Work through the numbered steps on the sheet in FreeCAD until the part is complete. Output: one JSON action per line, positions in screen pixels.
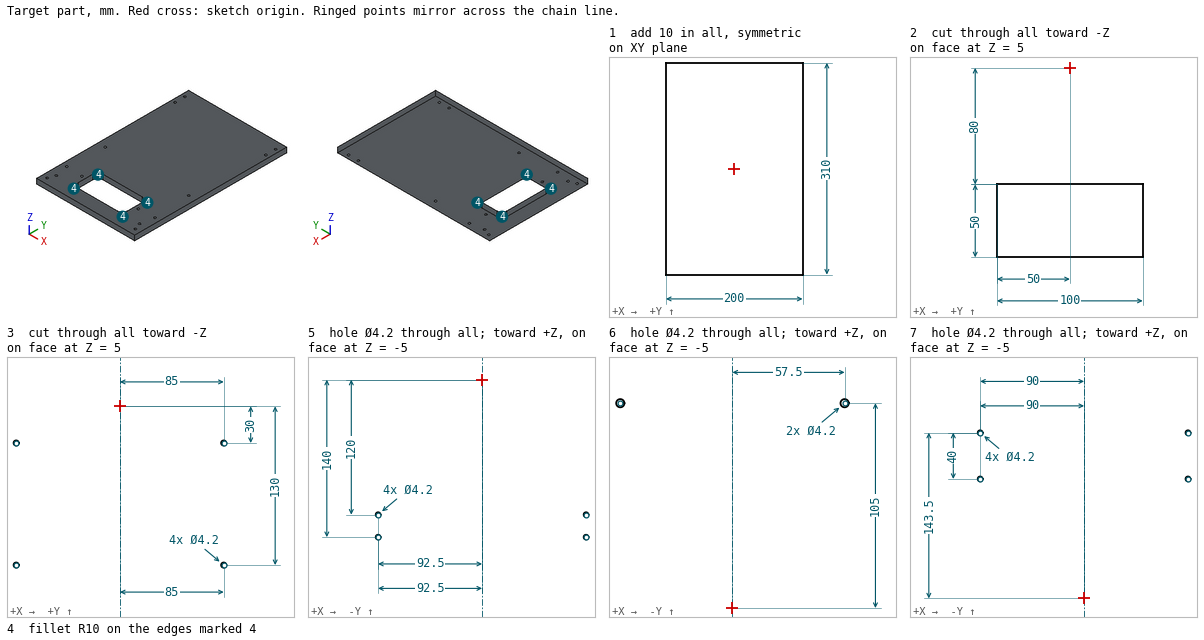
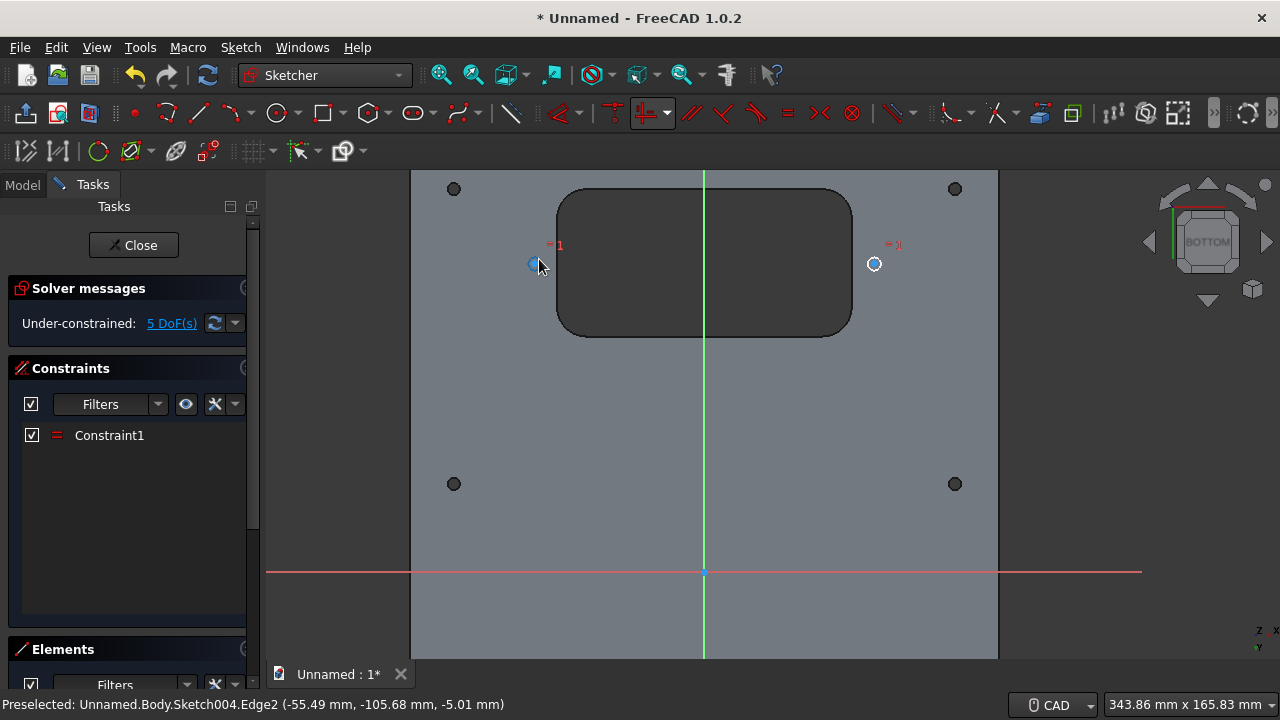
{"action": "left_click", "coordinate": [874, 264]}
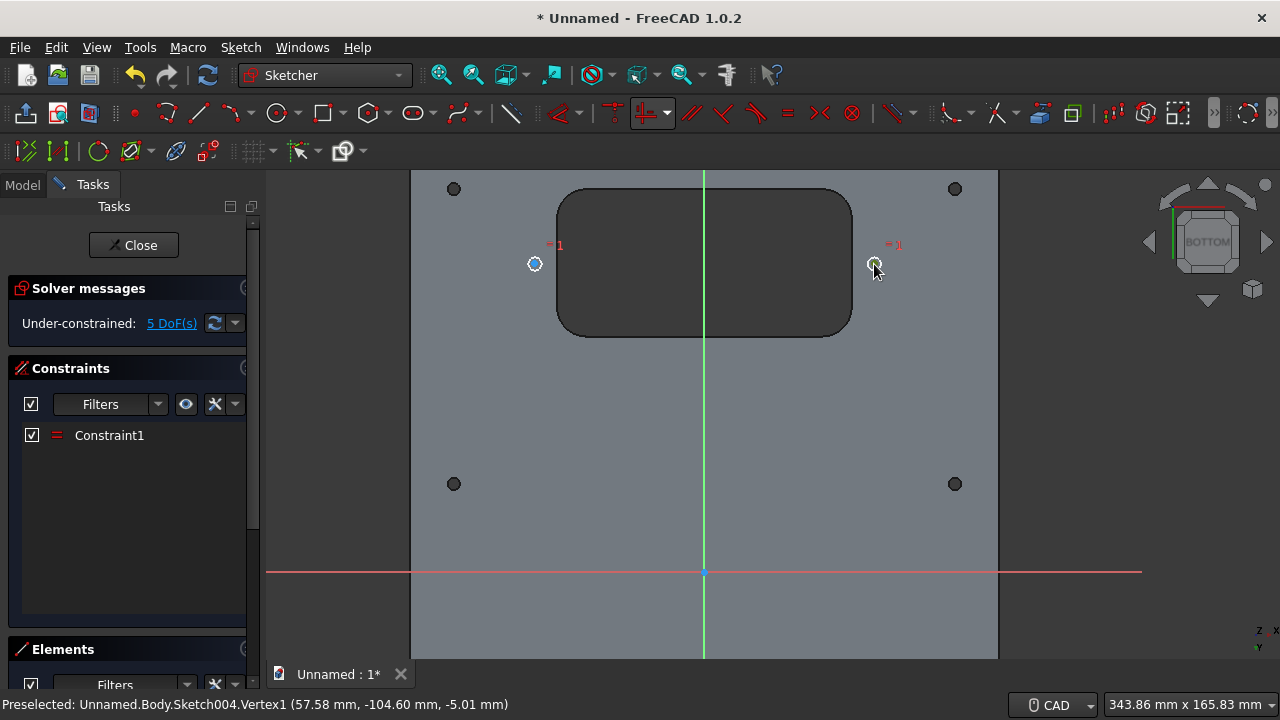
{"action": "left_click", "coordinate": [535, 264]}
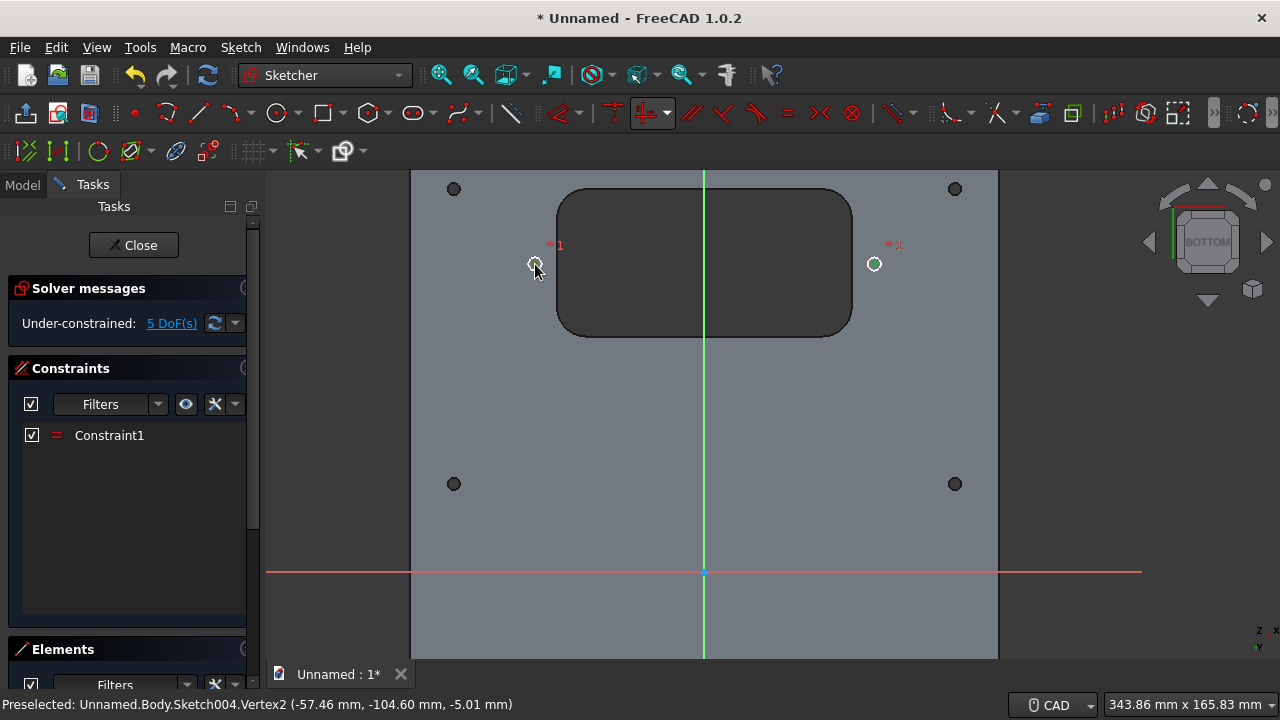
{"action": "left_click", "coordinate": [704, 538]}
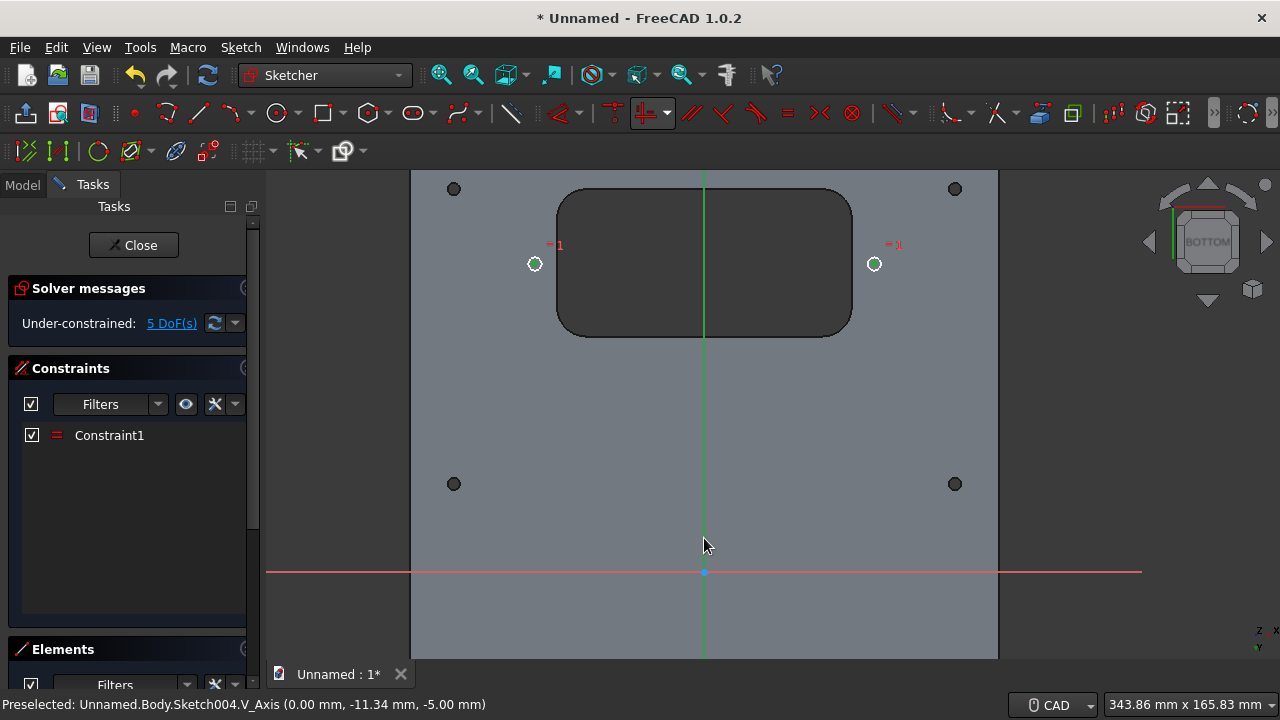
{"action": "left_click", "coordinate": [820, 114]}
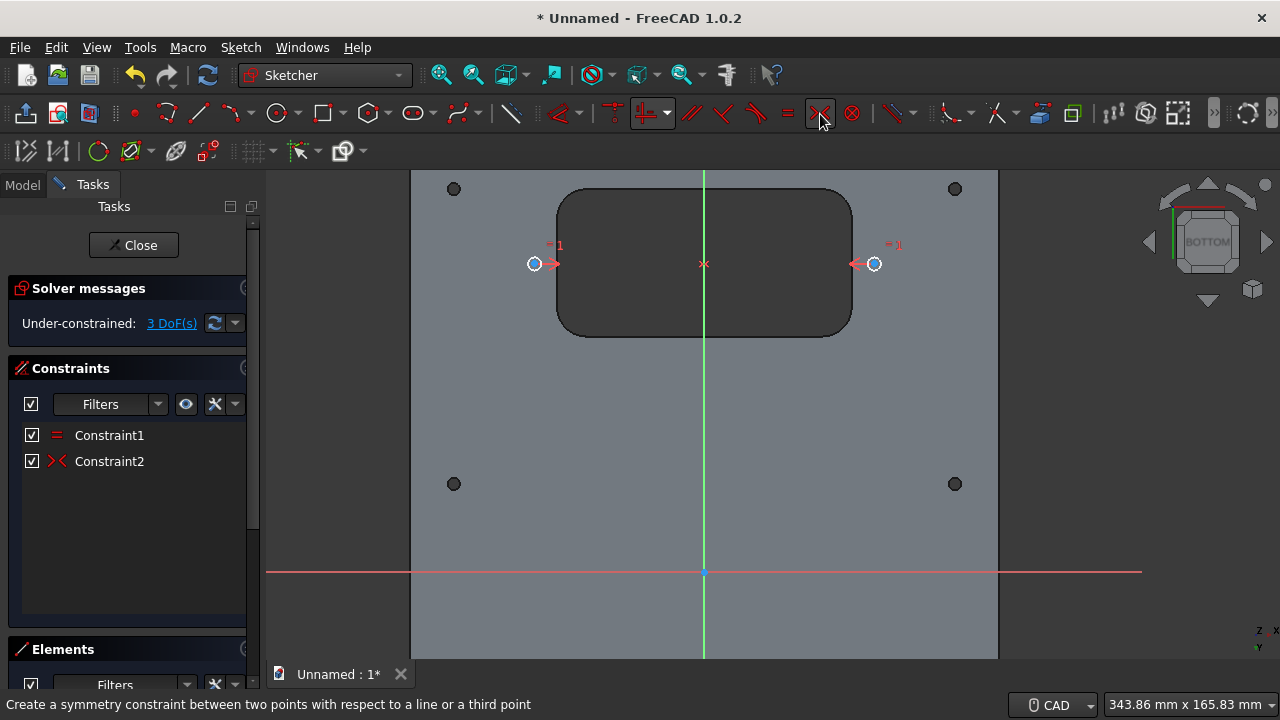
{"action": "left_click", "coordinate": [558, 114]}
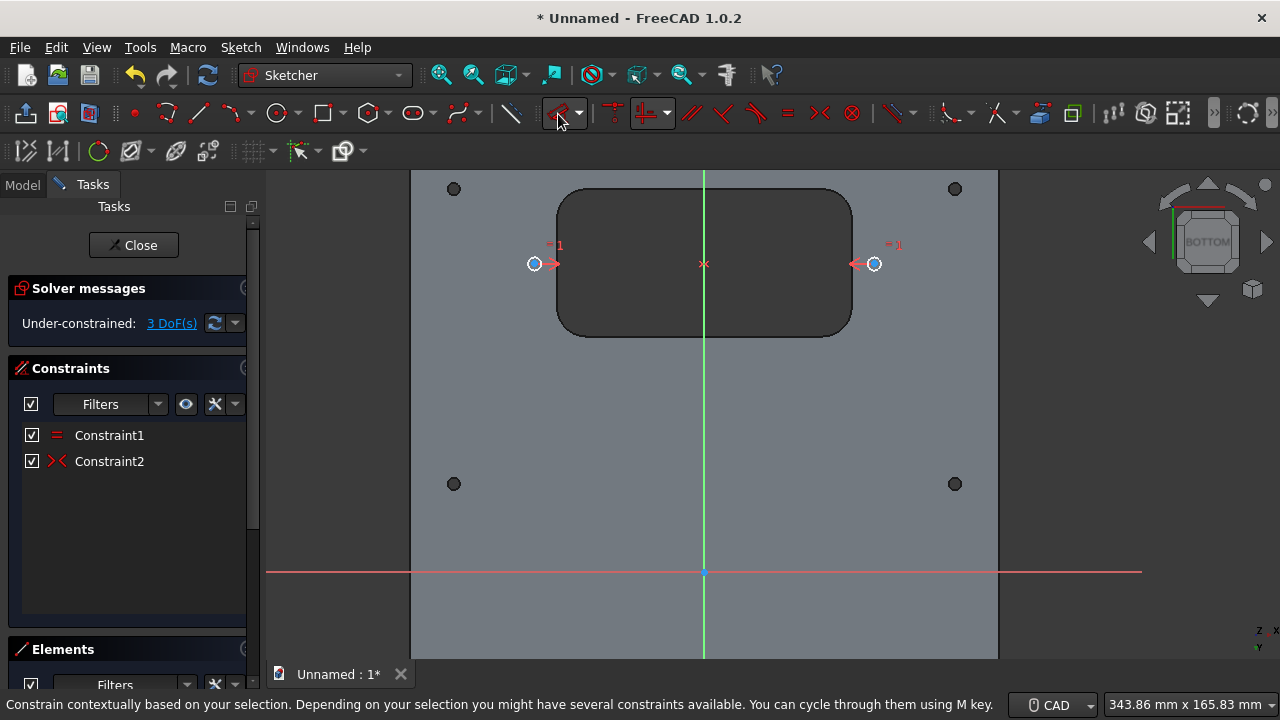
{"action": "scroll", "coordinate": [879, 259], "scroll_direction": "up", "scroll_amount": 6}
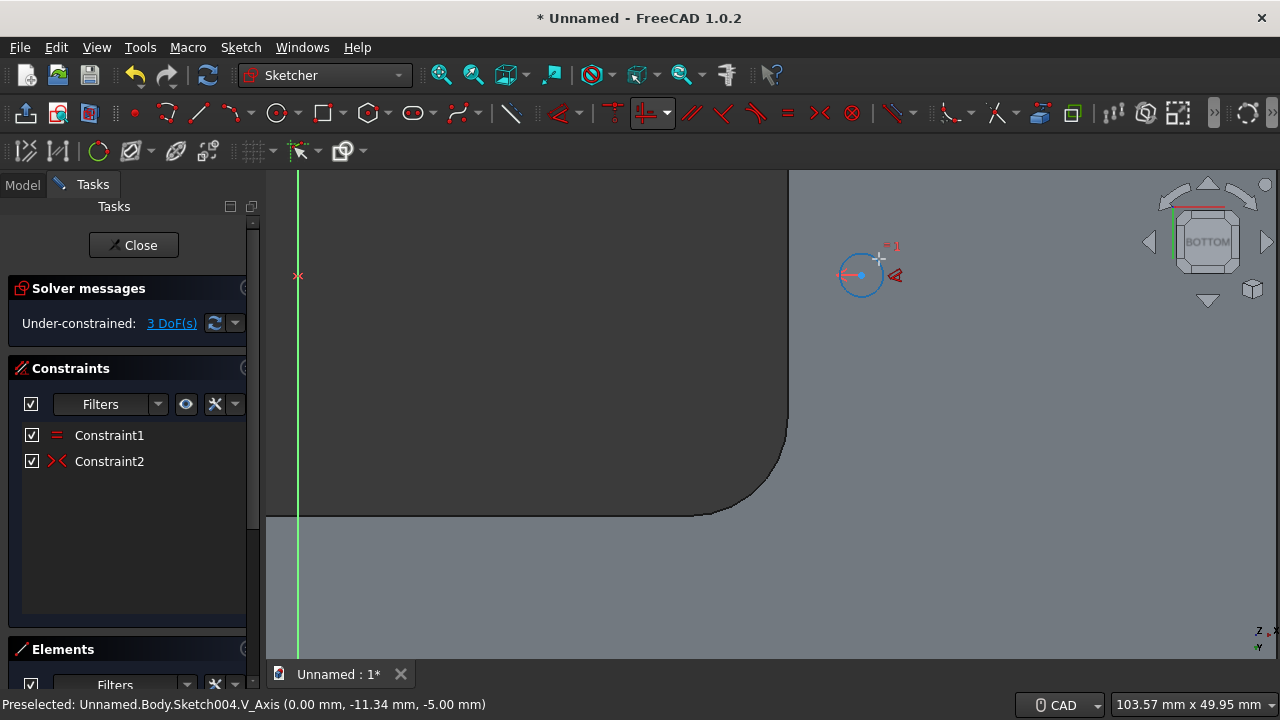
{"action": "left_click", "coordinate": [877, 260]}
{"action": "left_click", "coordinate": [900, 238]}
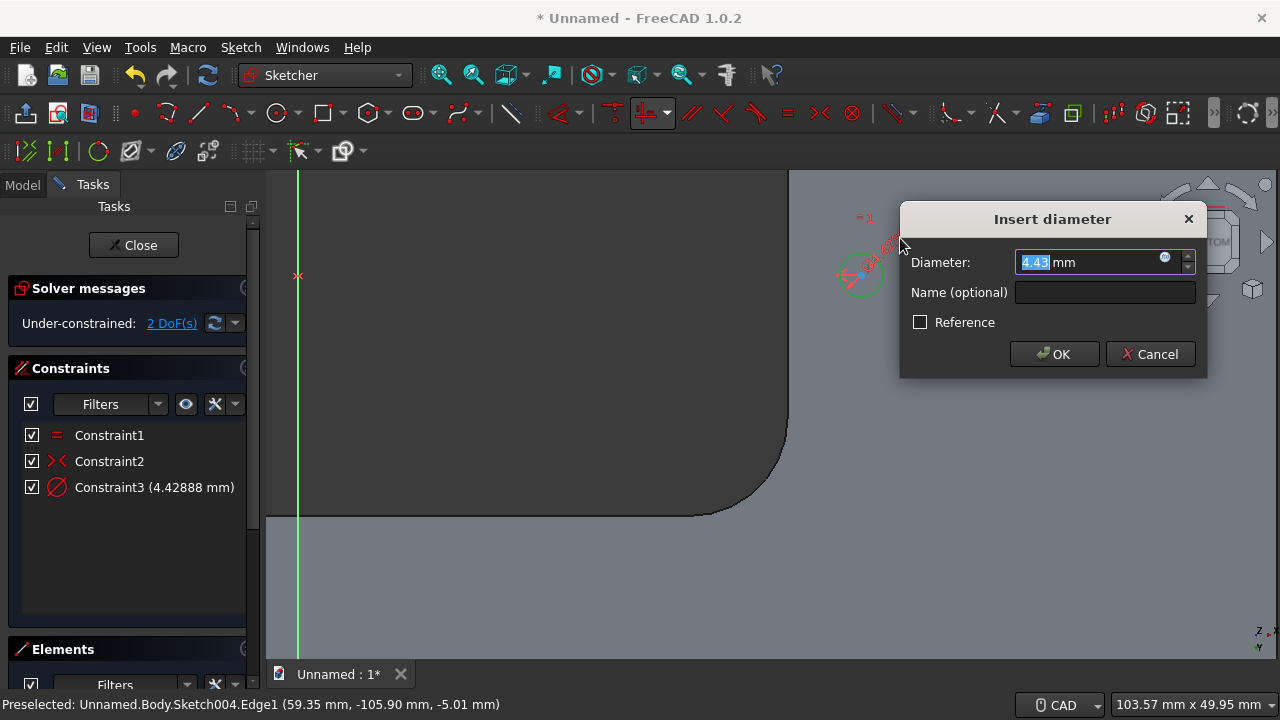
{"action": "type", "text": "4.2"}
{"action": "key", "text": "Return"}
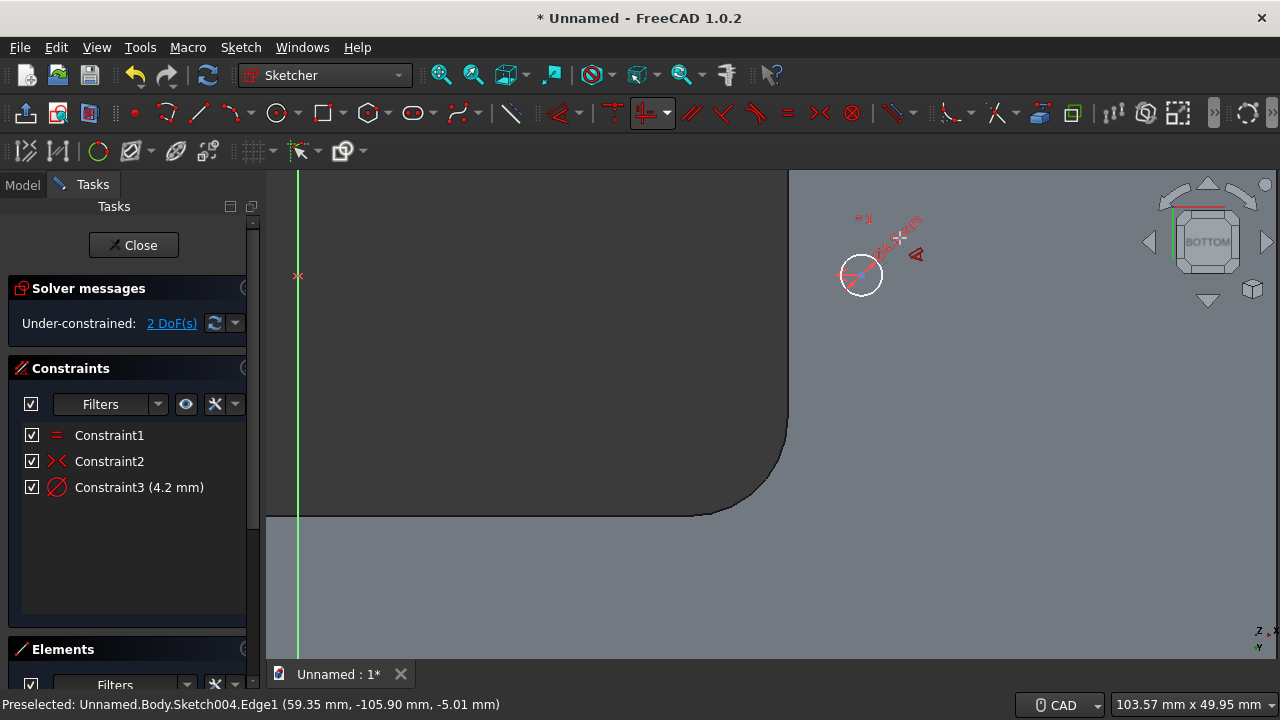
{"action": "left_click", "coordinate": [862, 275]}
{"action": "left_click", "coordinate": [896, 453]}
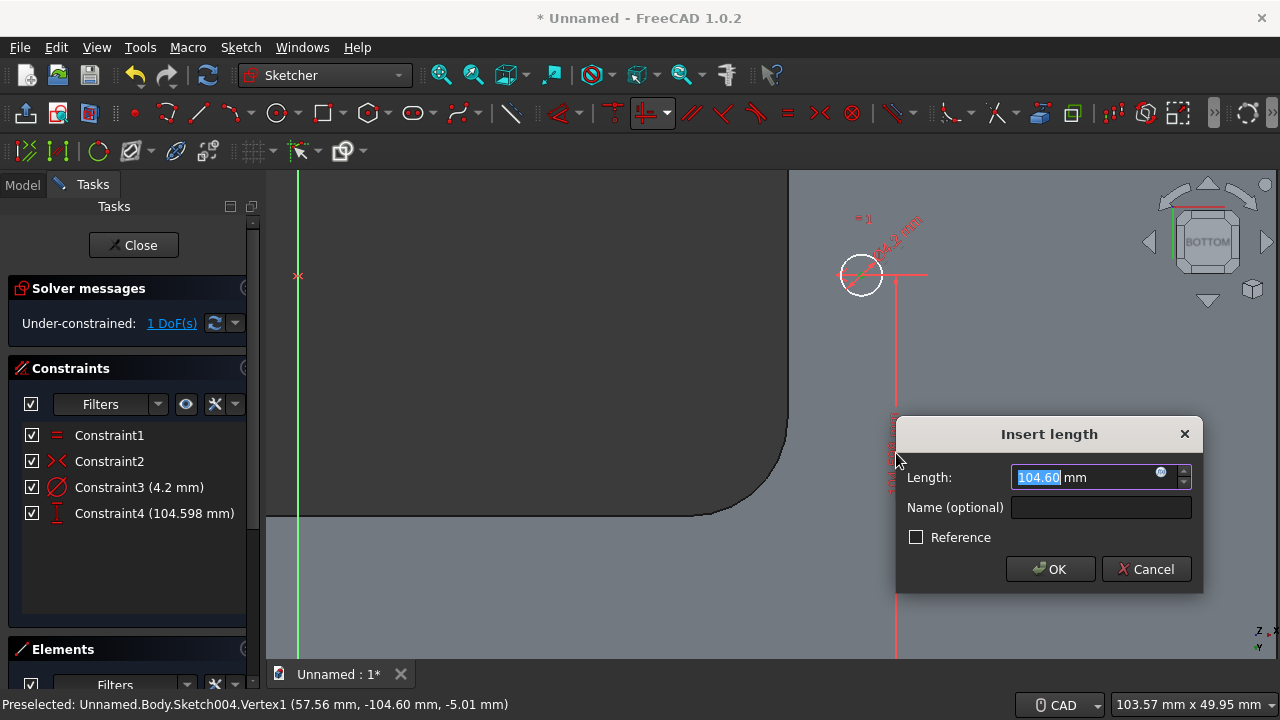
{"action": "type", "text": "105"}
{"action": "key", "text": "Return"}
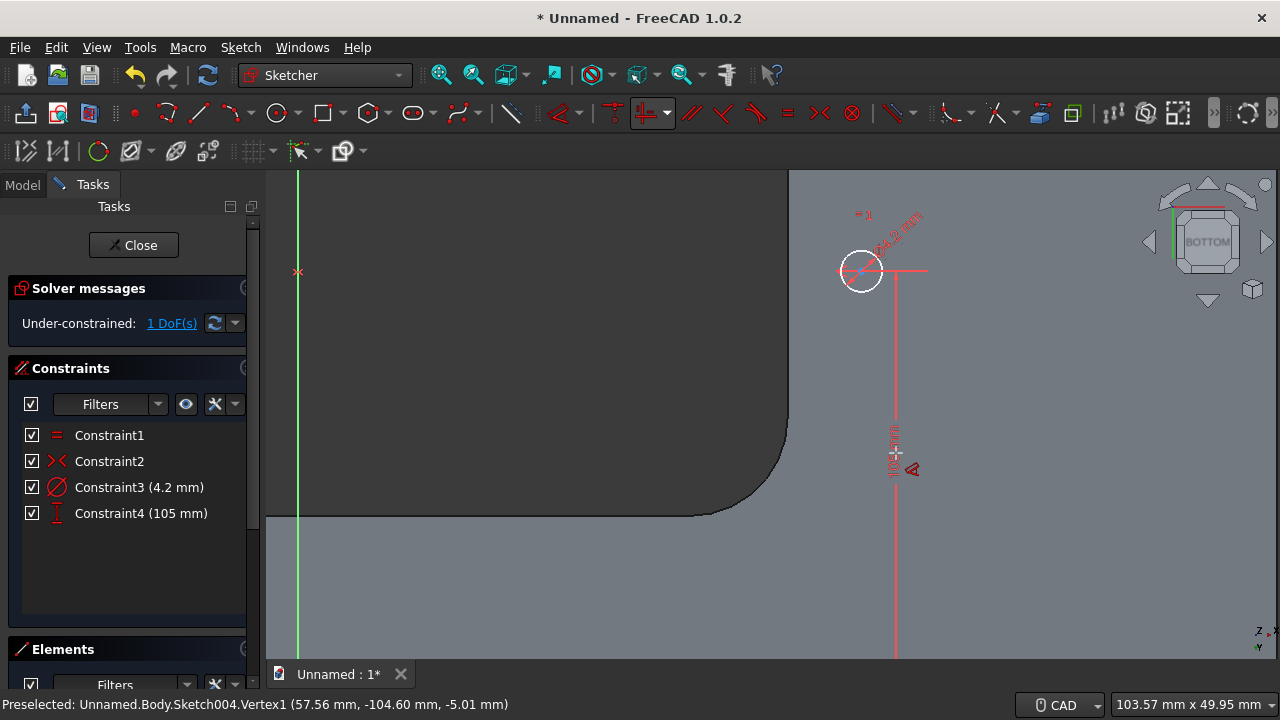
{"action": "left_click", "coordinate": [862, 271]}
{"action": "left_click", "coordinate": [580, 237]}